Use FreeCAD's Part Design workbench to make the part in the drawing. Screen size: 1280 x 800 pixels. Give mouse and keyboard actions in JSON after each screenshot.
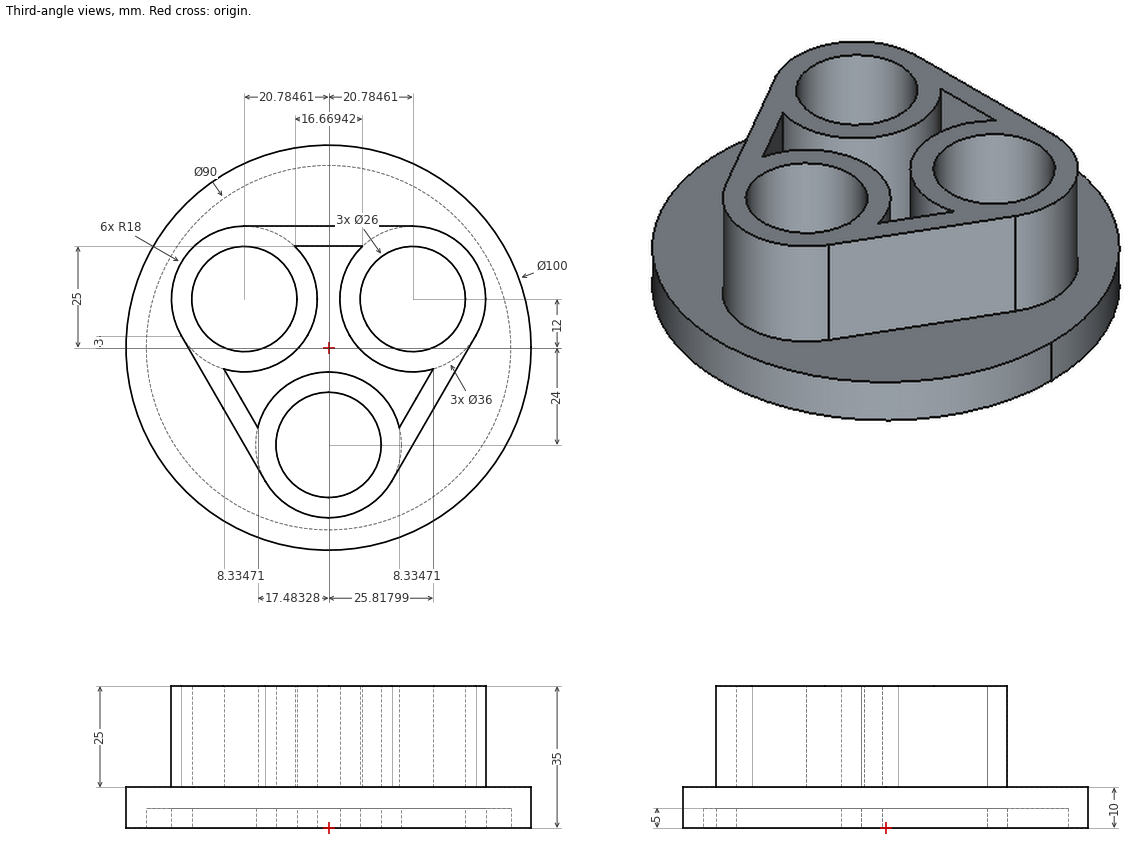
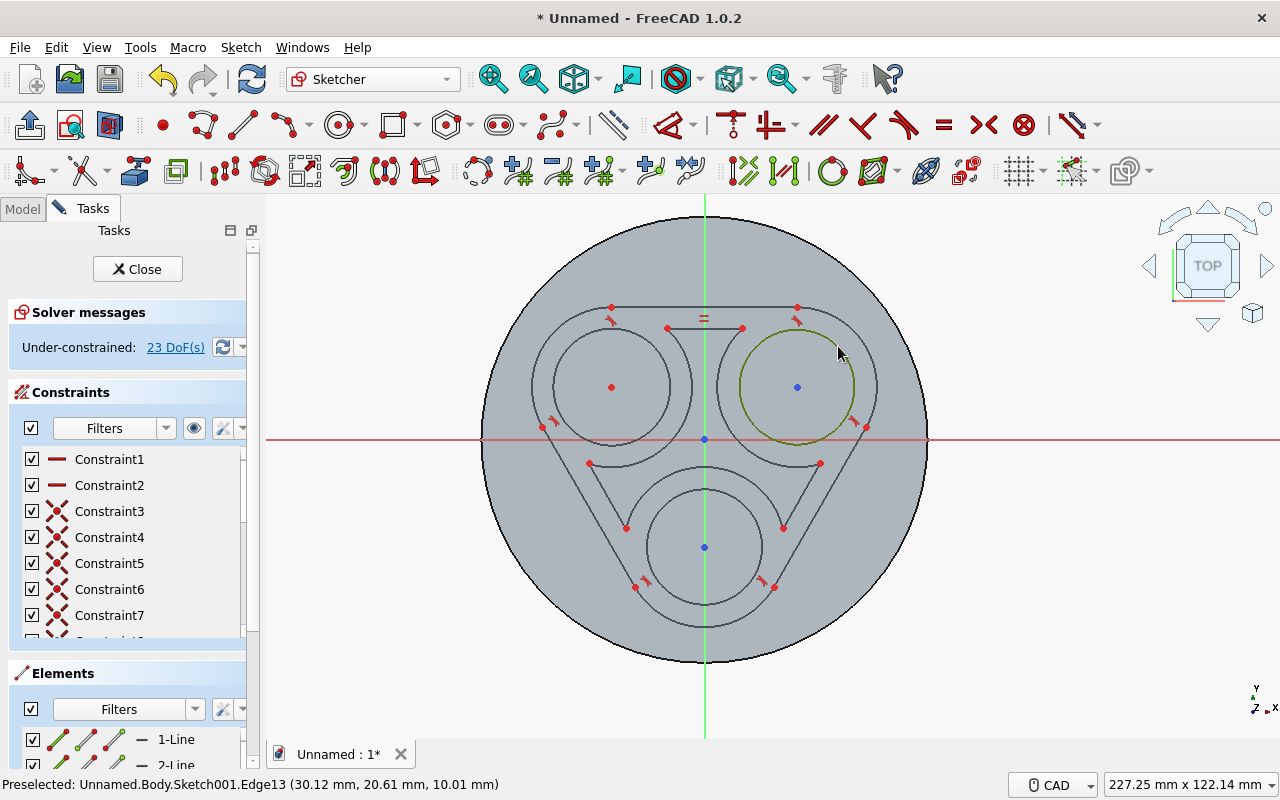
{"action": "left_click", "coordinate": [717, 386]}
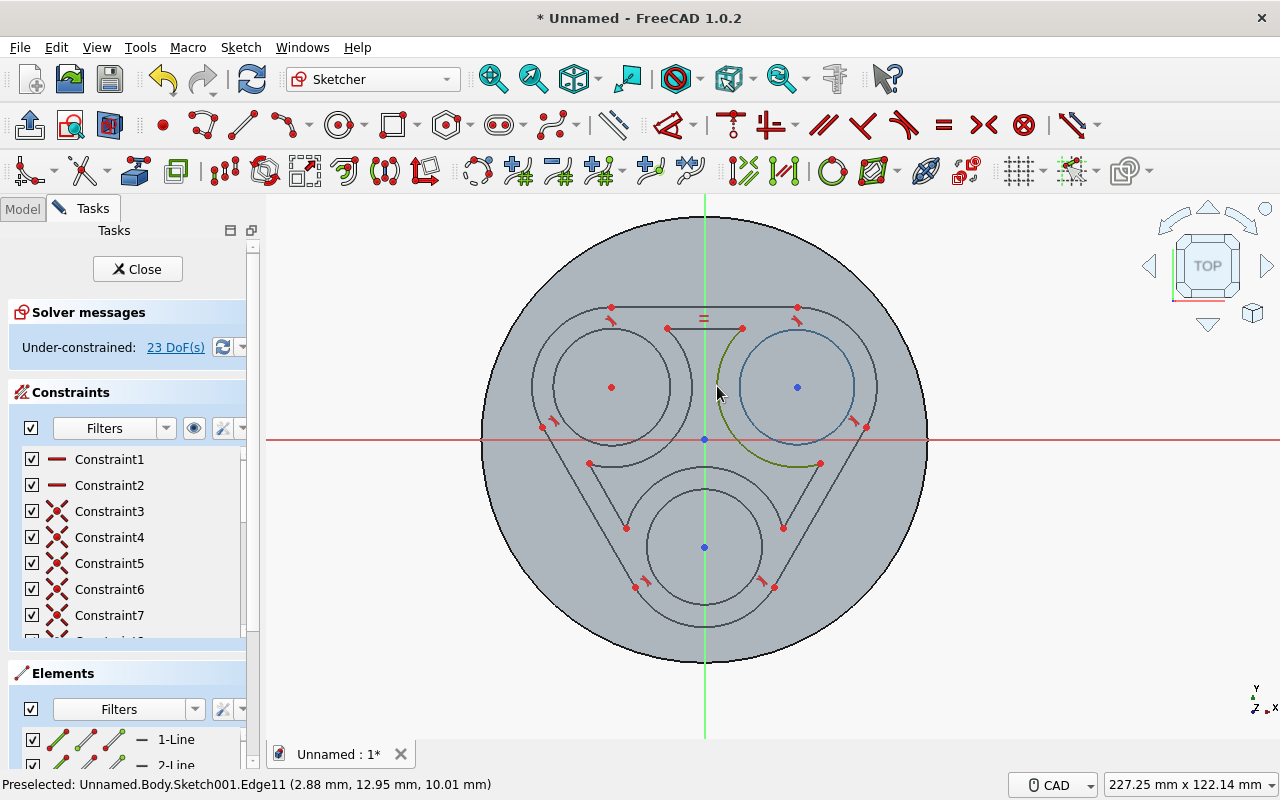
{"action": "left_click", "coordinate": [732, 126]}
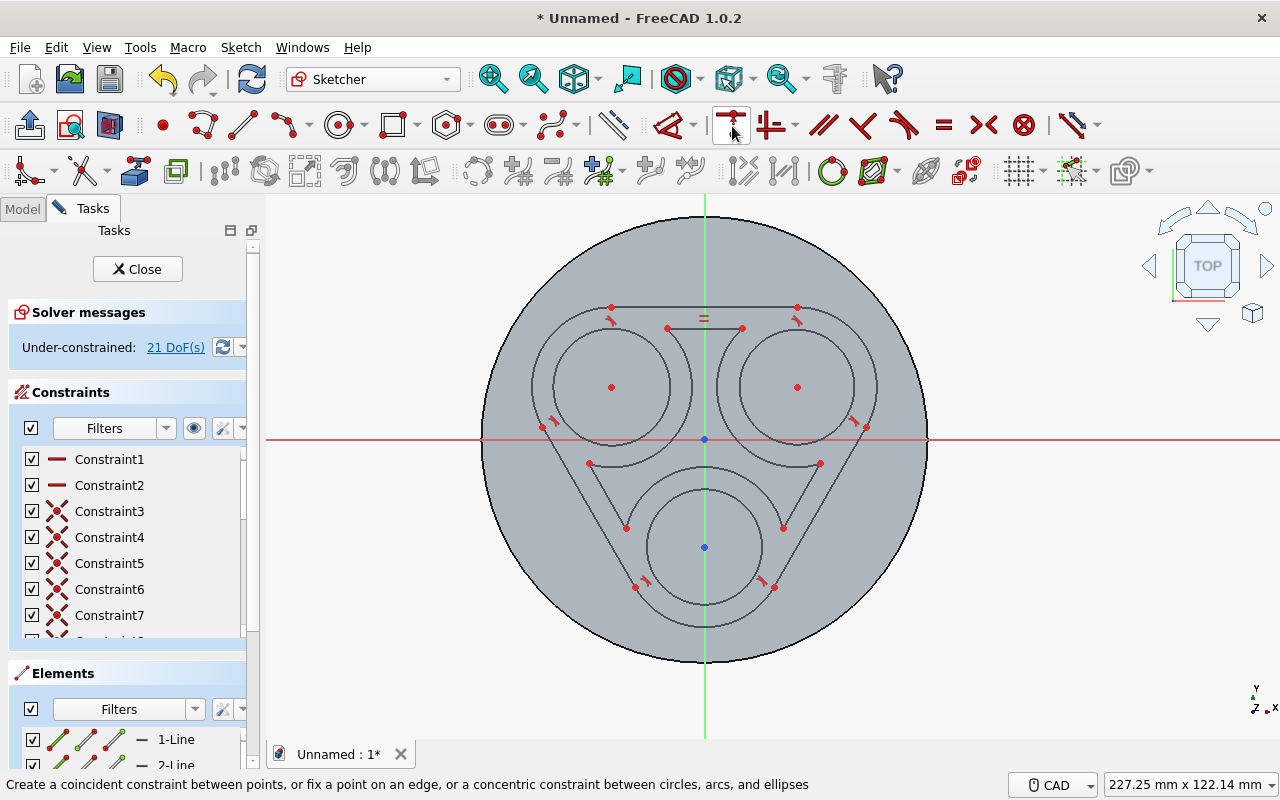
{"action": "left_click", "coordinate": [745, 506]}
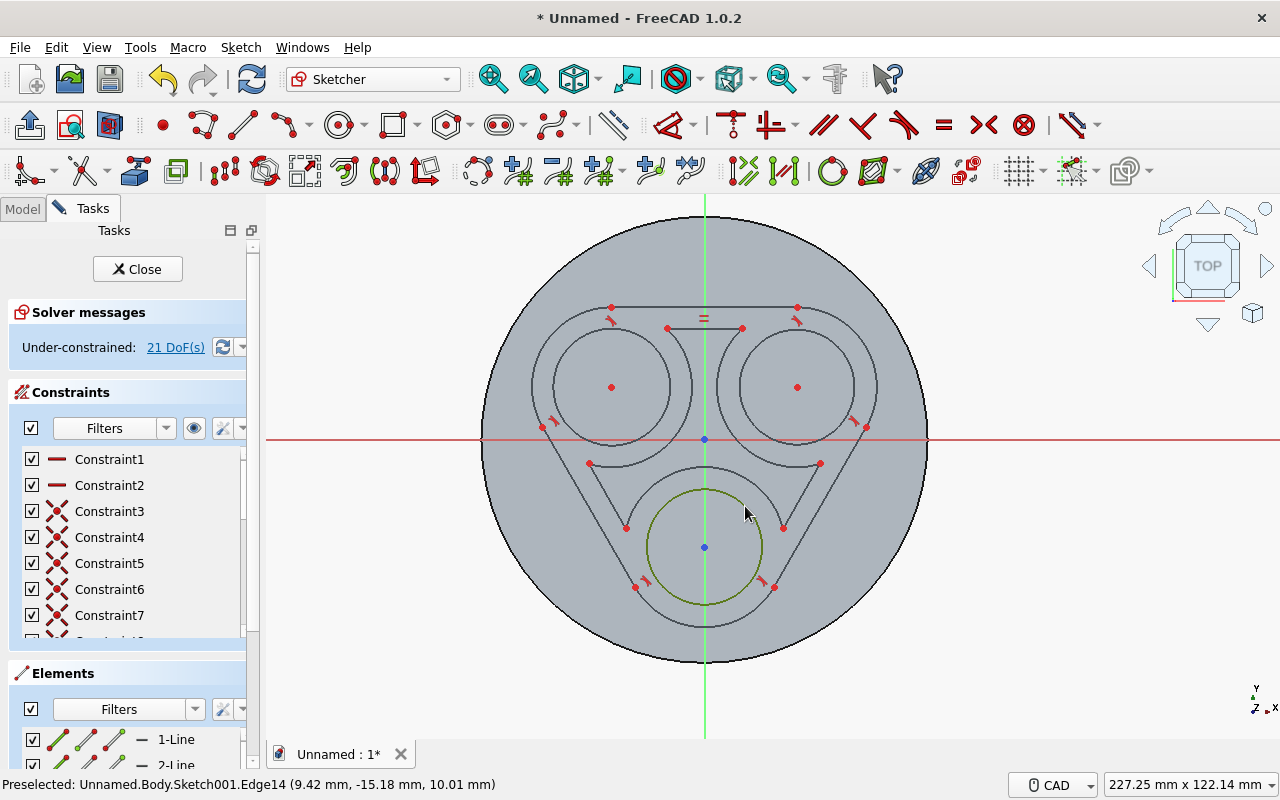
{"action": "left_click", "coordinate": [746, 478]}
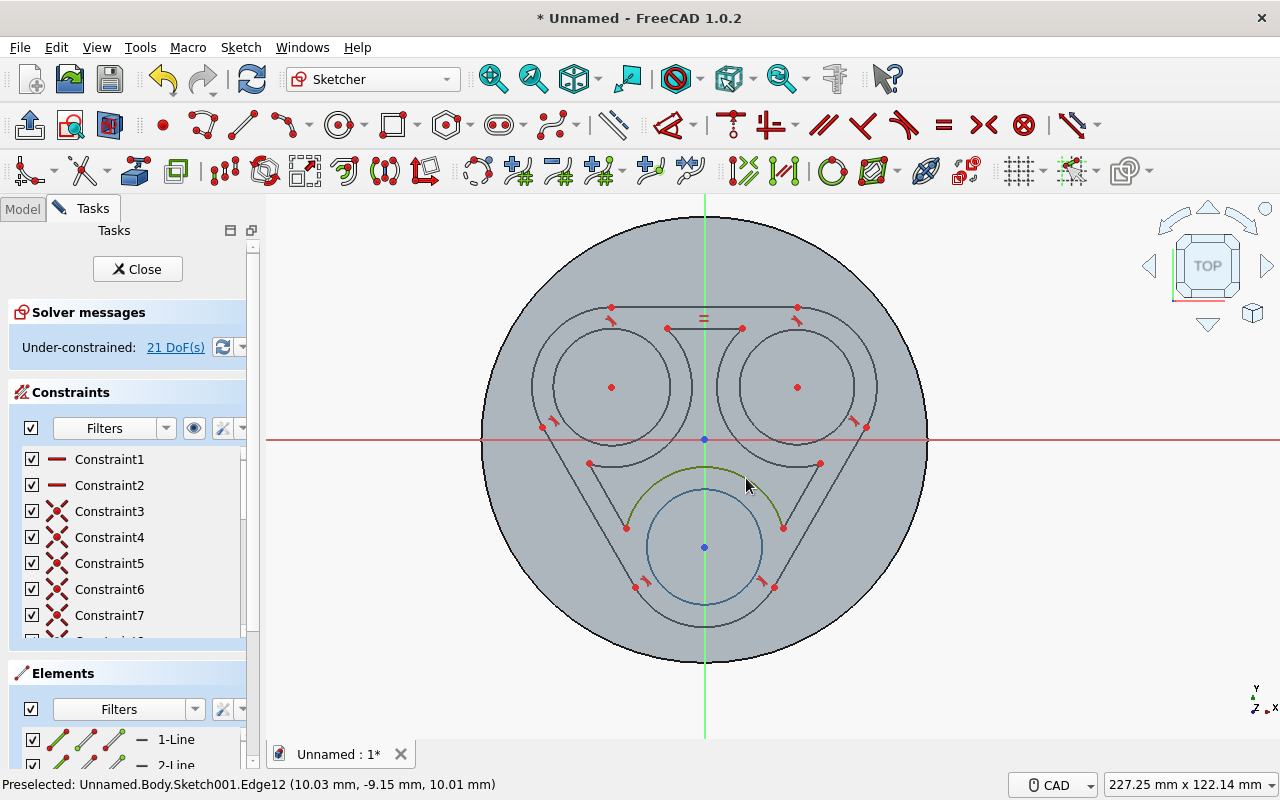
{"action": "left_click", "coordinate": [732, 126]}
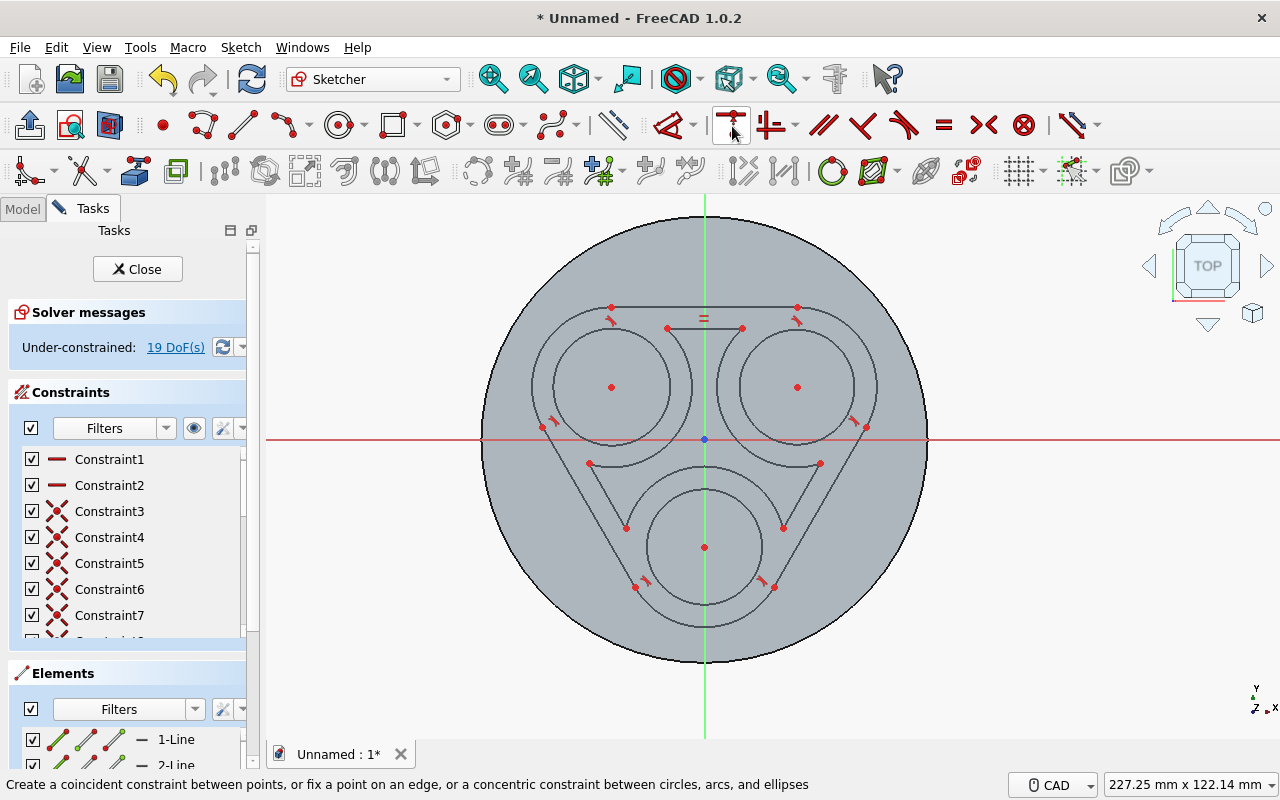
{"action": "left_click", "coordinate": [672, 620]}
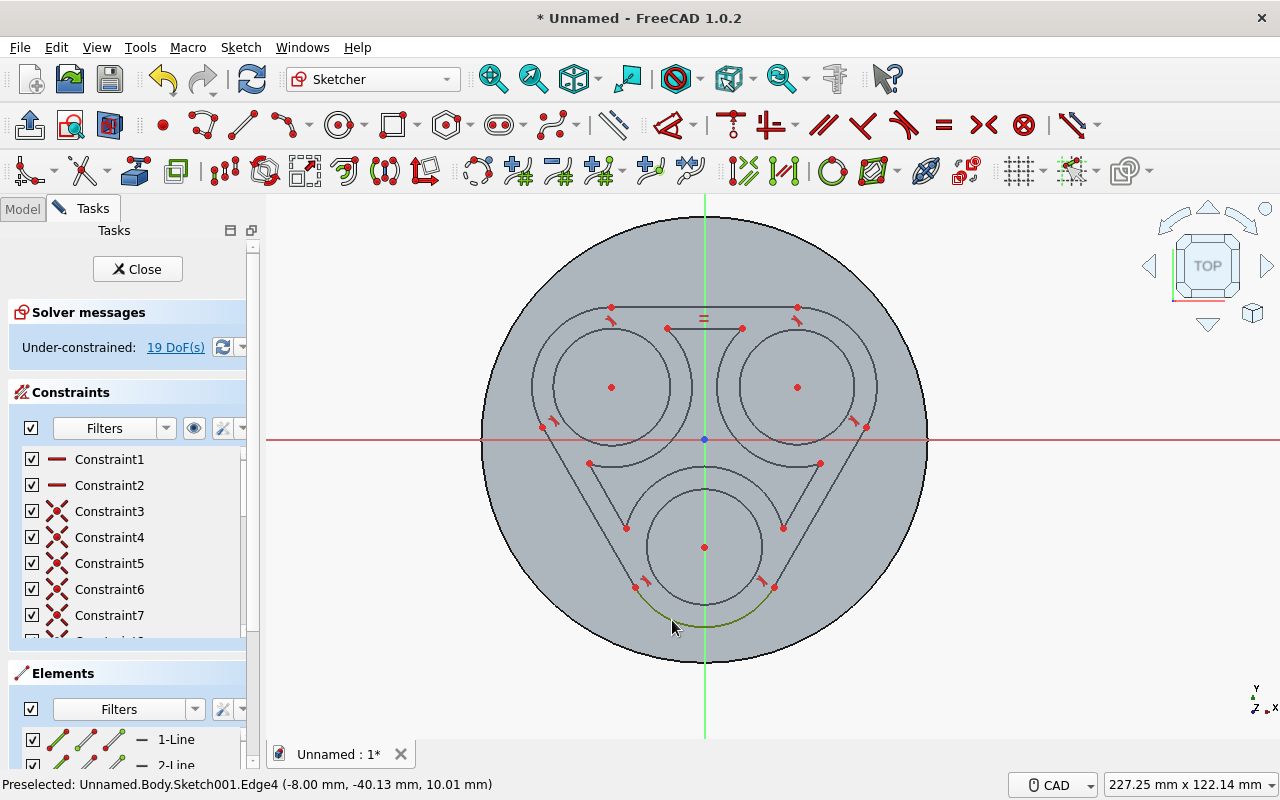
{"action": "left_click", "coordinate": [876, 379]}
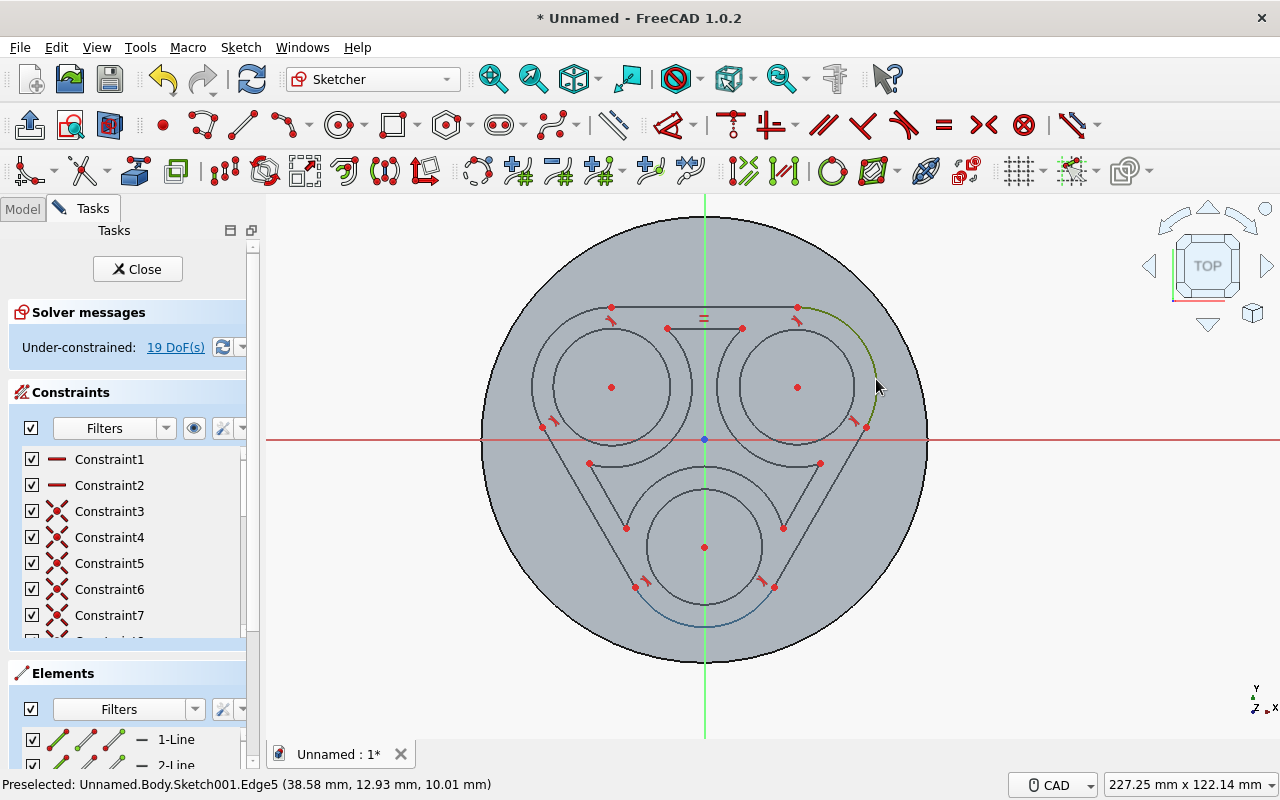
{"action": "left_click", "coordinate": [565, 323]}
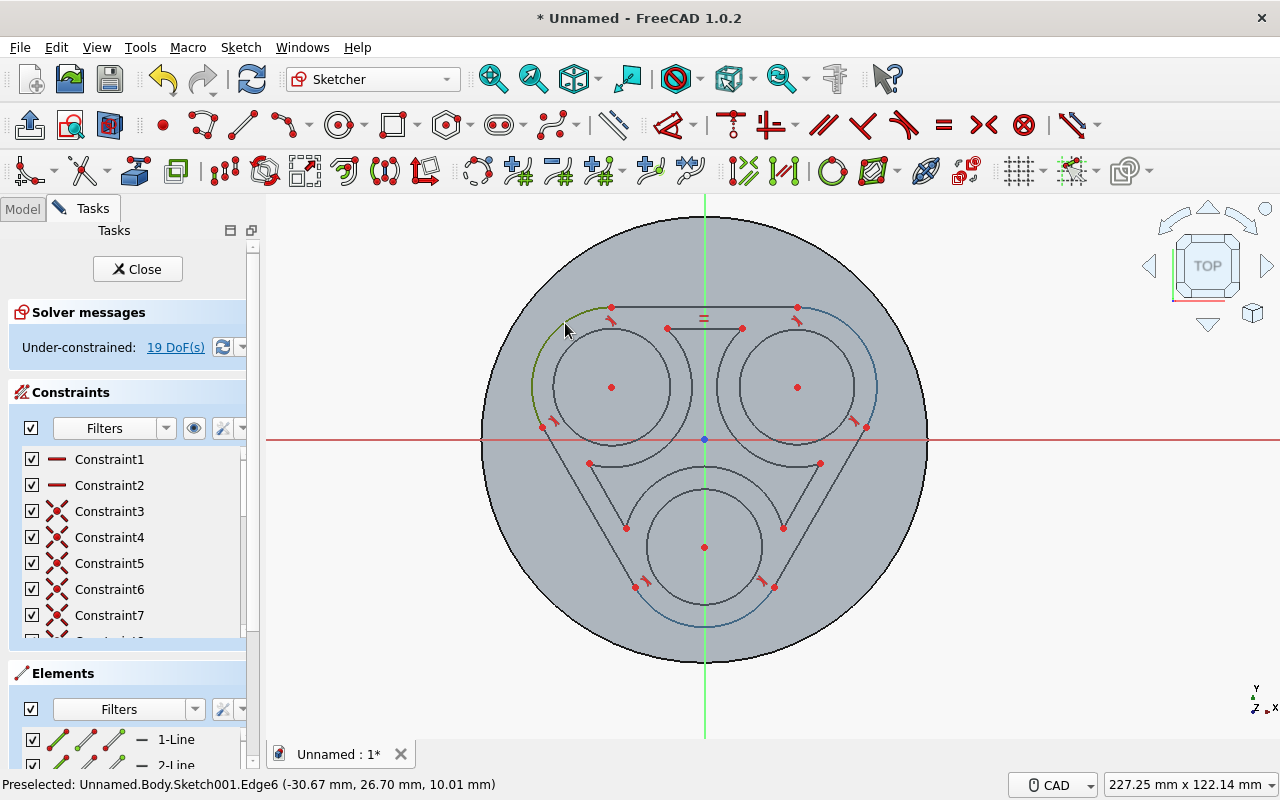
{"action": "left_click", "coordinate": [651, 457]}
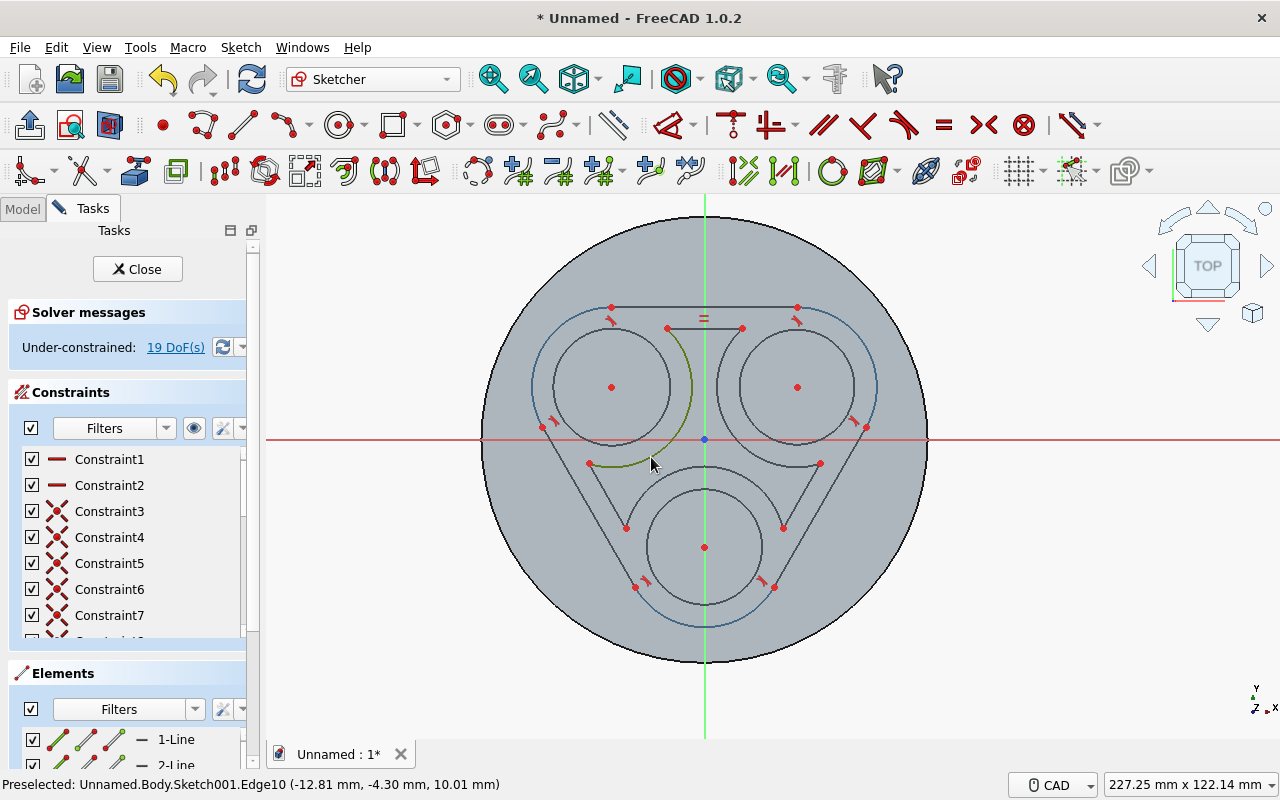
{"action": "left_click", "coordinate": [717, 386]}